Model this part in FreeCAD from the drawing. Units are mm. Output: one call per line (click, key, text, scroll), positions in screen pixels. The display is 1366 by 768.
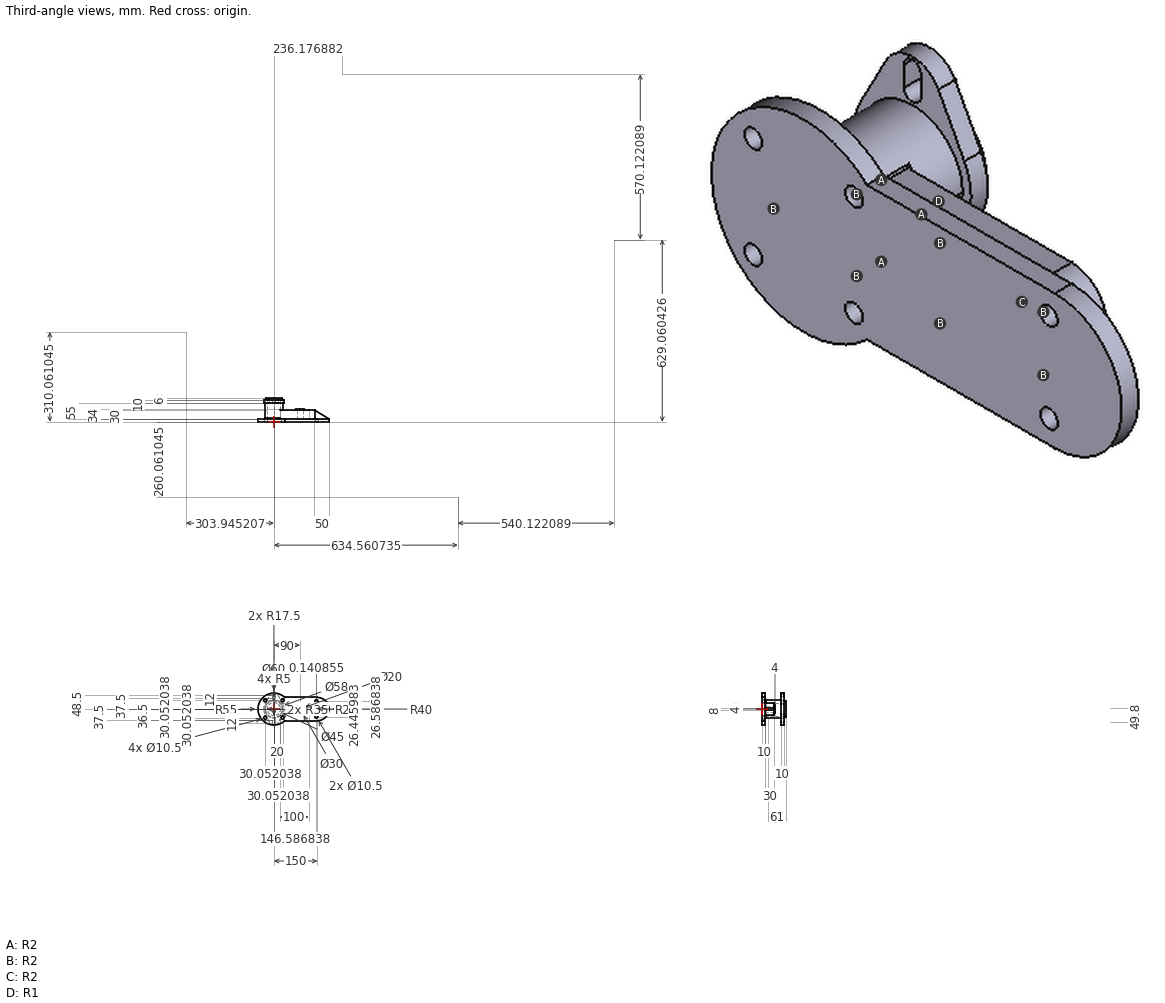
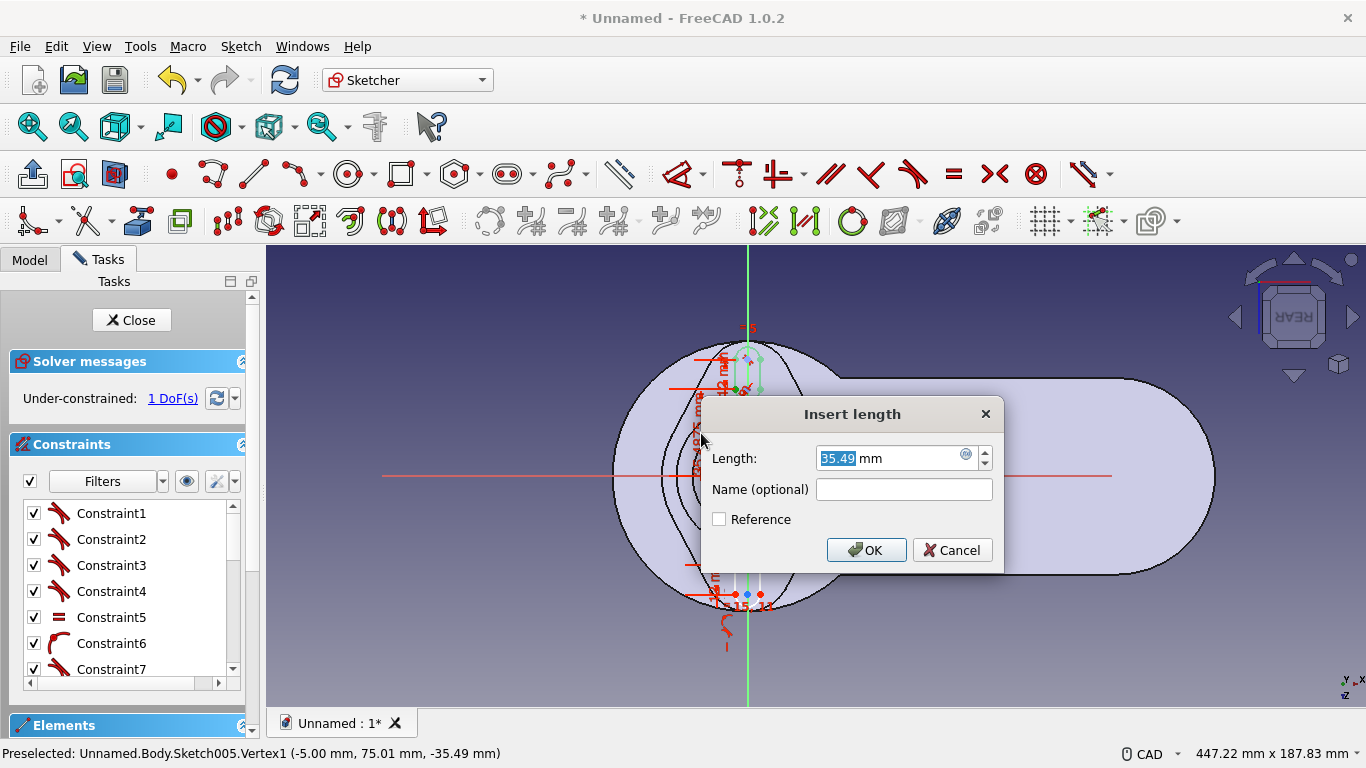
text(36.5)
key(Return)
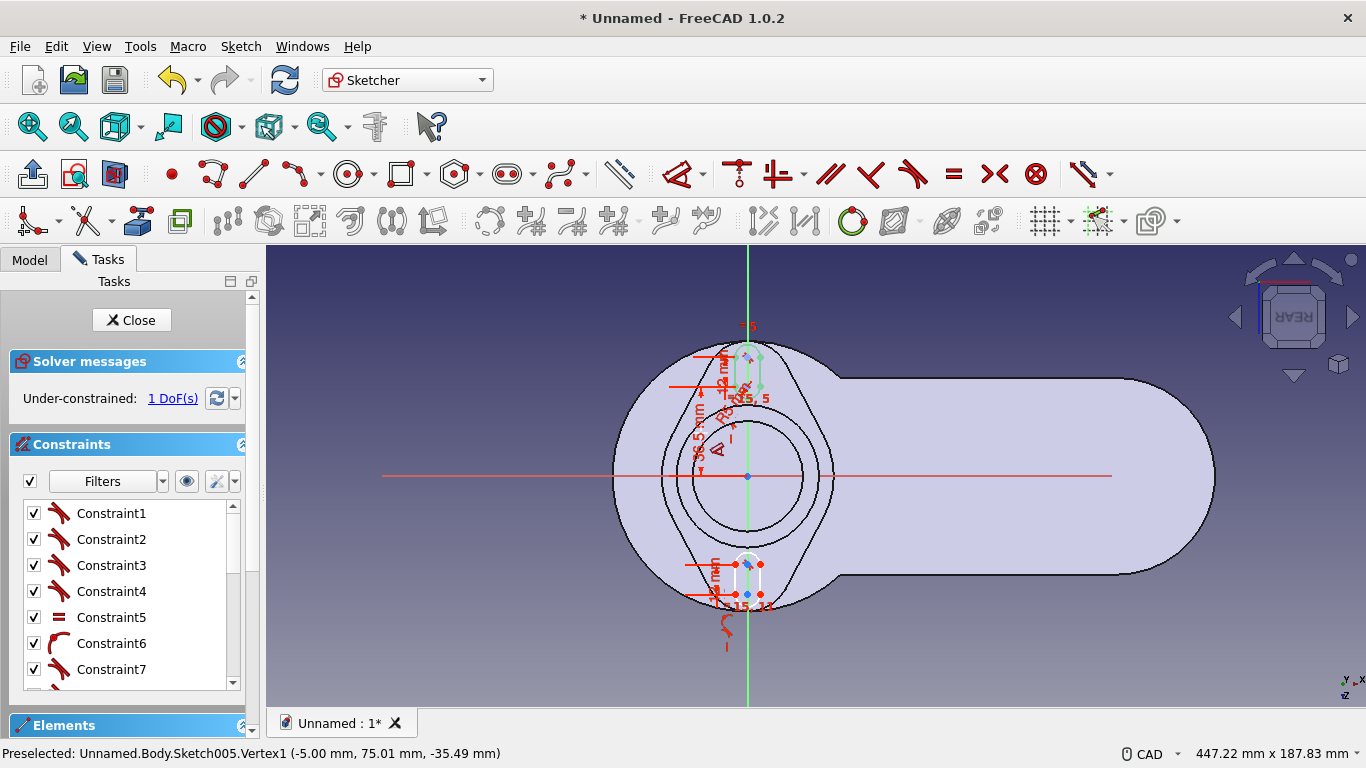
click(735, 595)
click(701, 535)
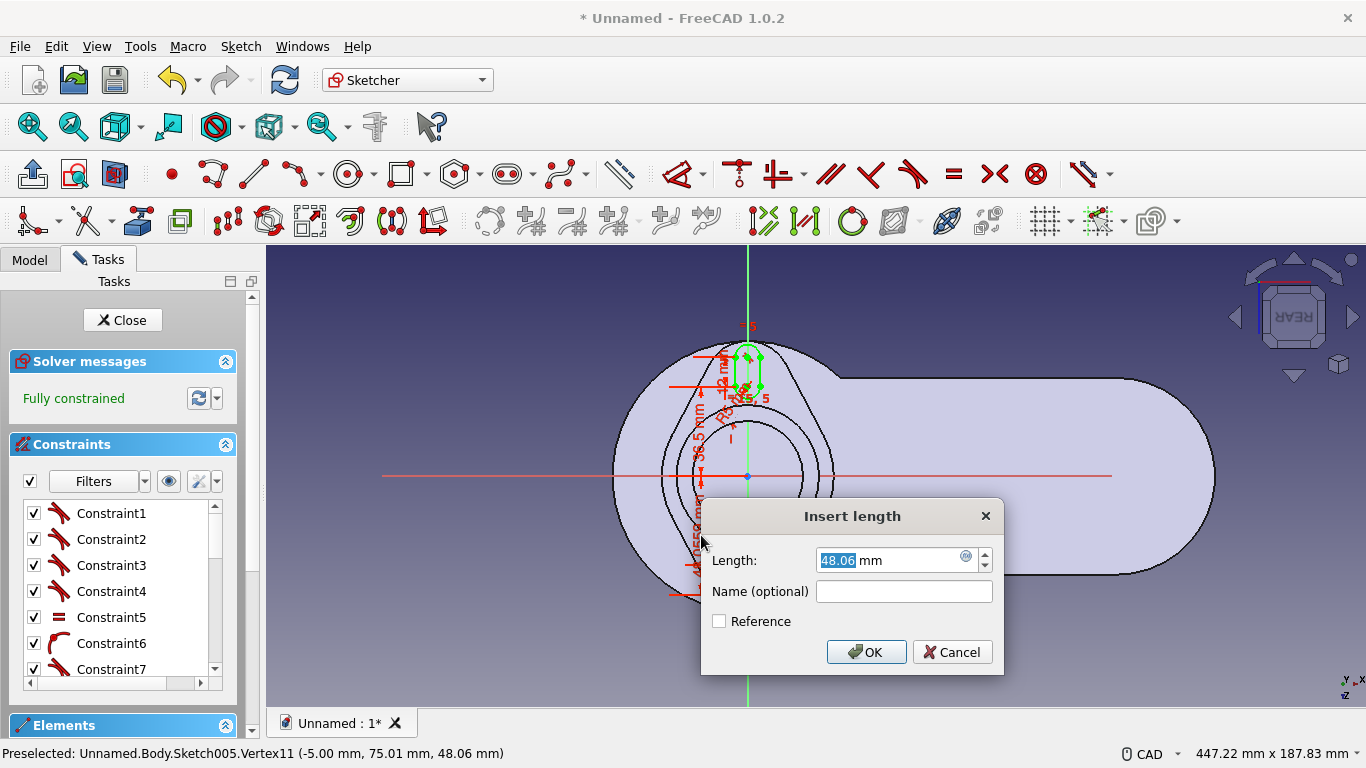
text(48.5)
key(Return)
key(Escape)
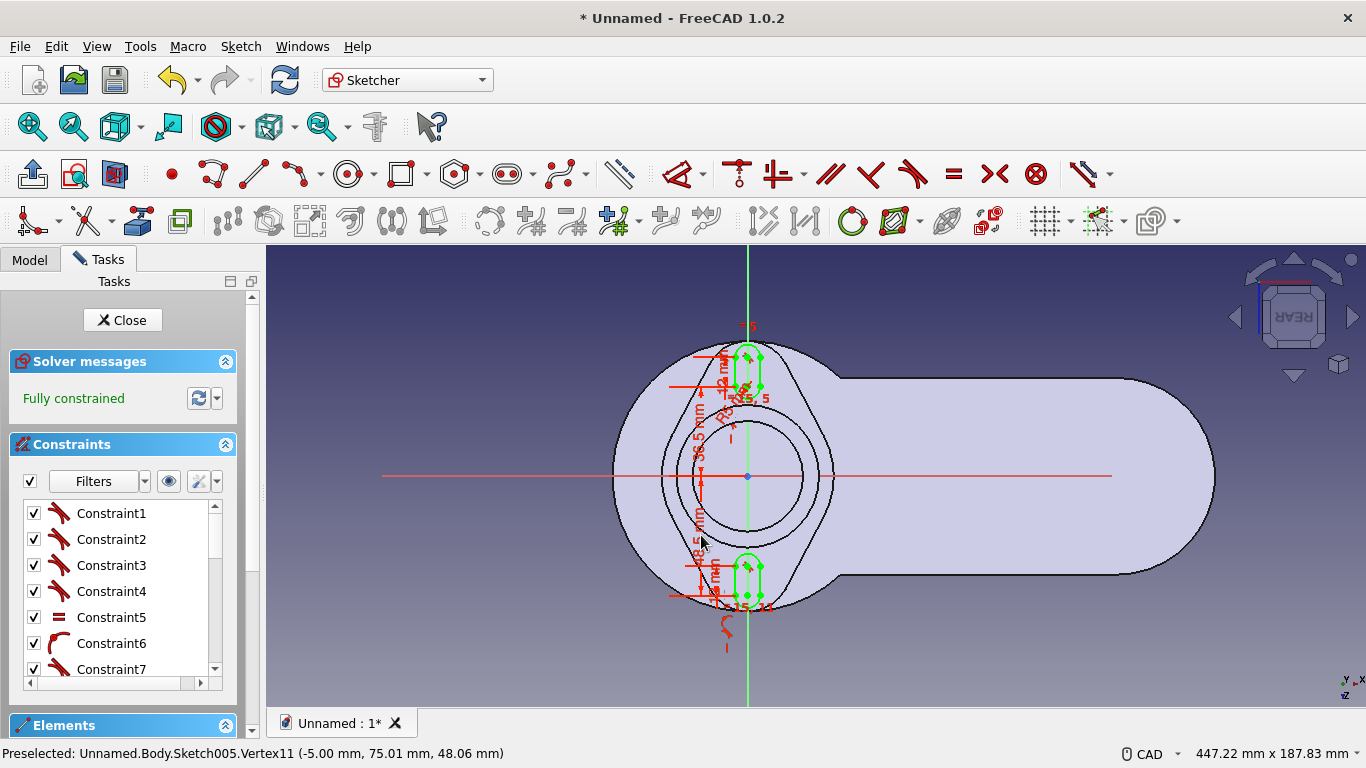
click(123, 320)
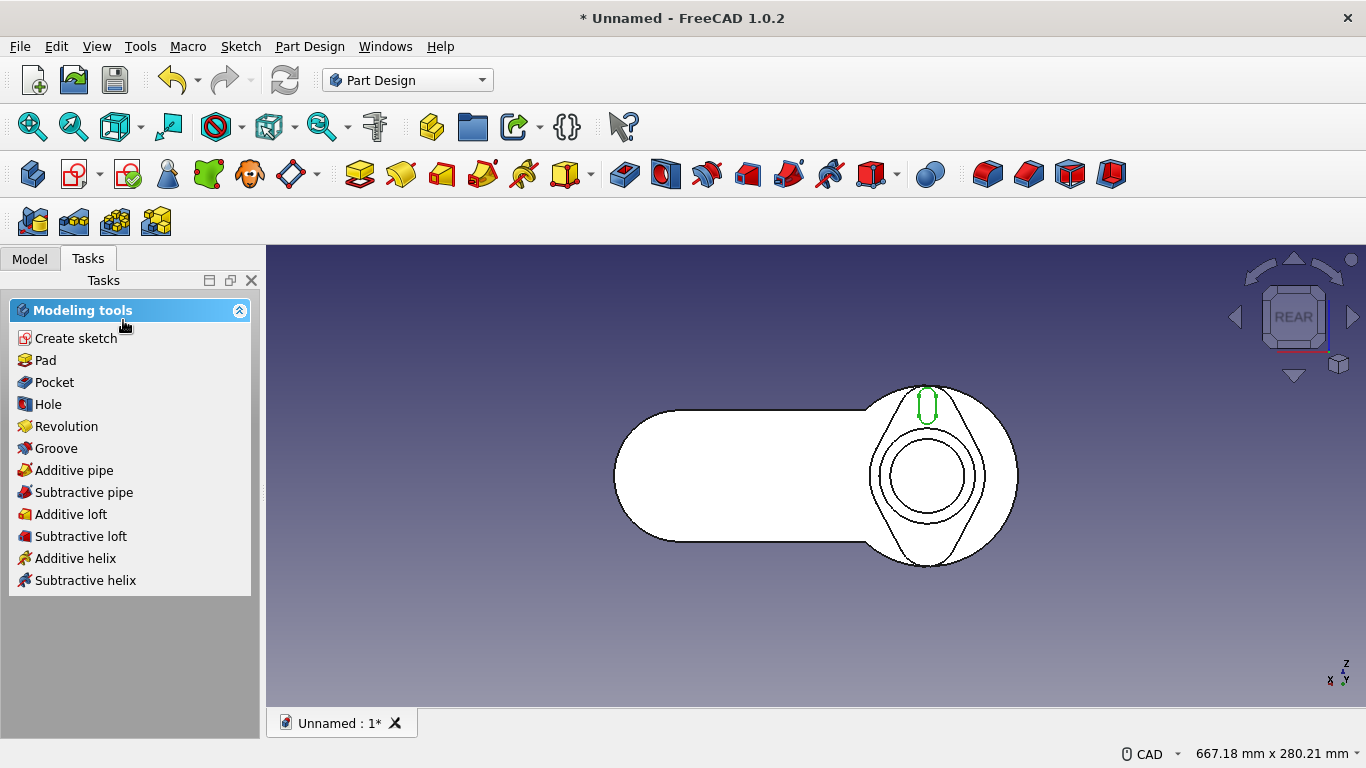
click(625, 174)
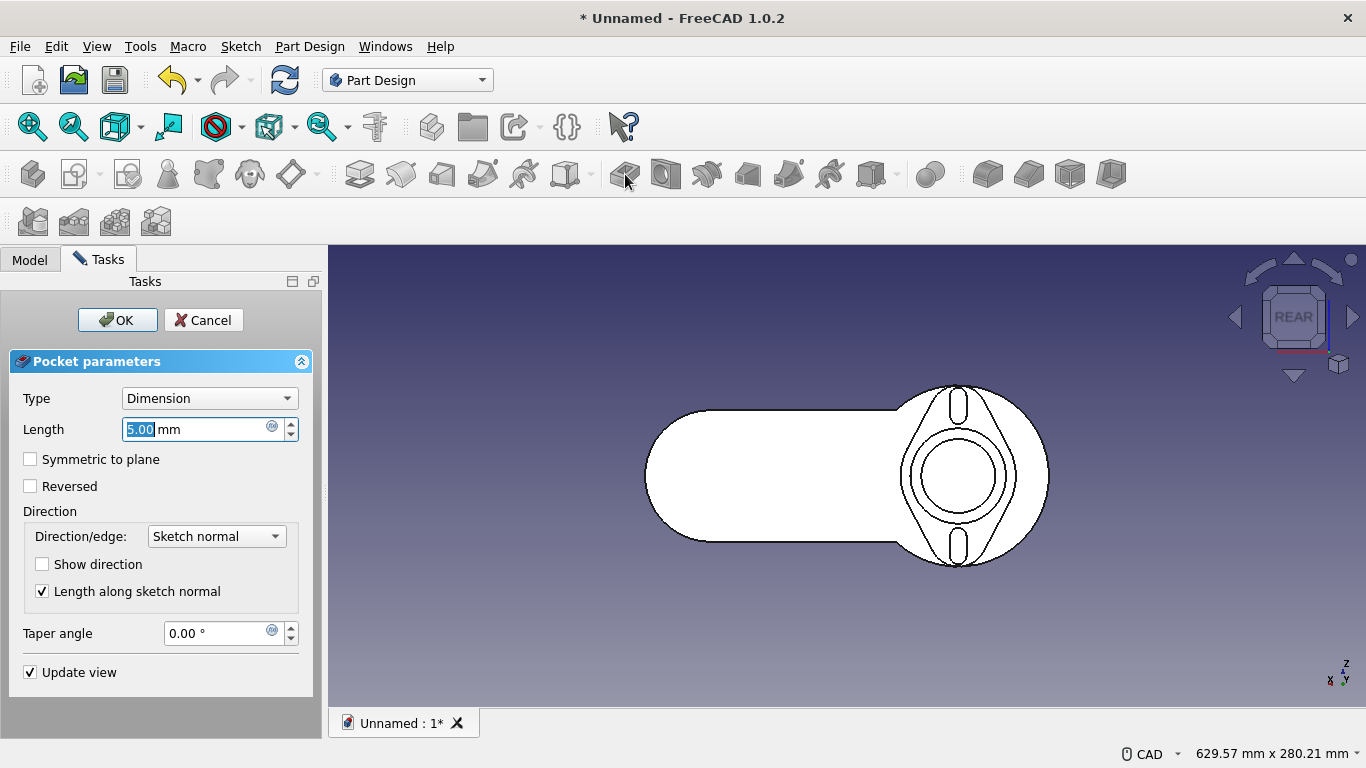
text(10)
key(Tab)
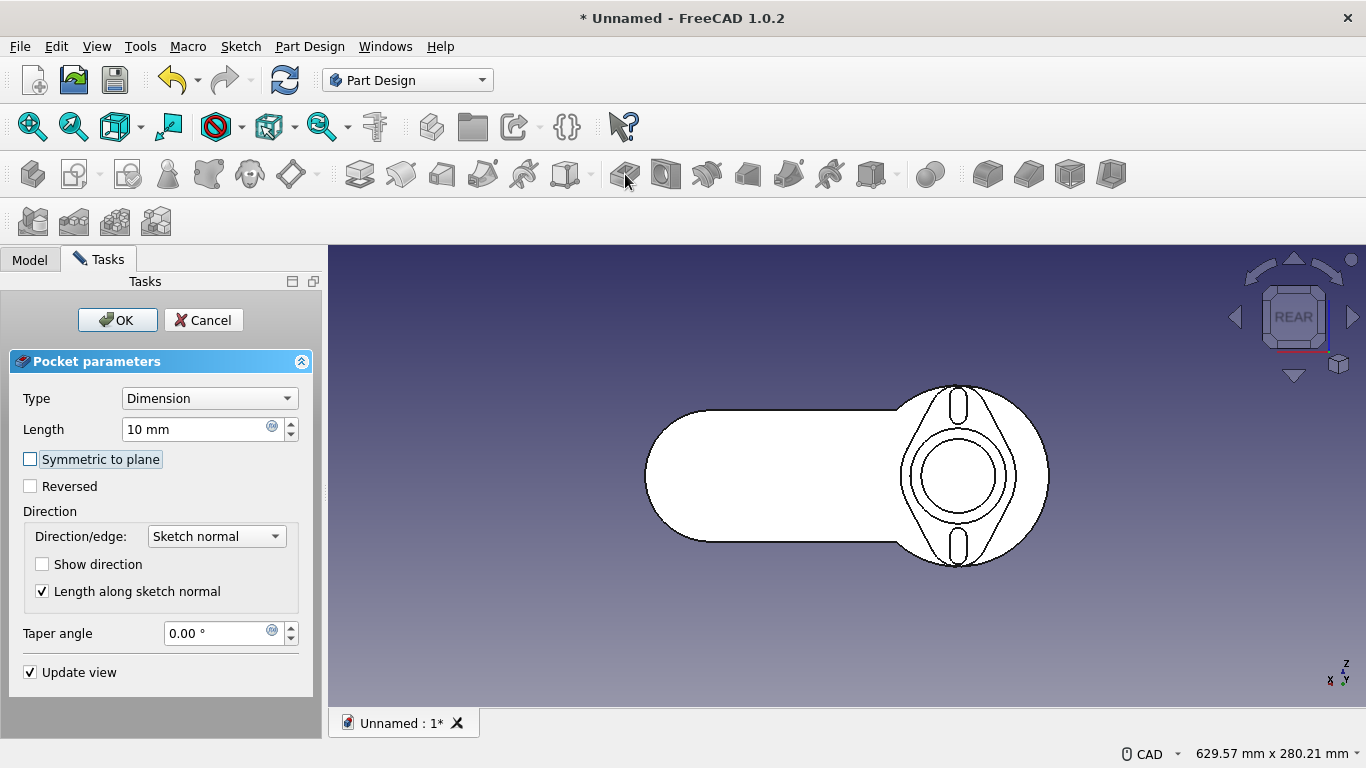
click(118, 320)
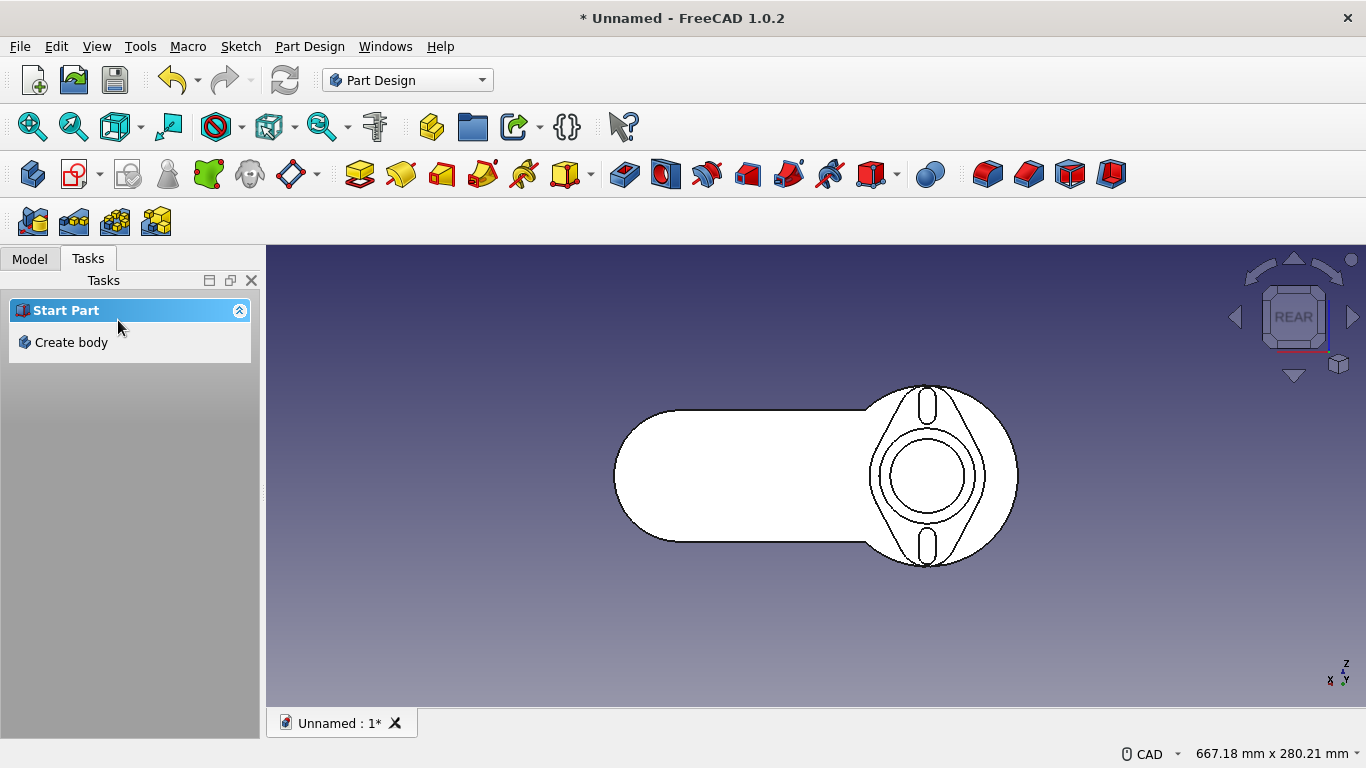
click(33, 128)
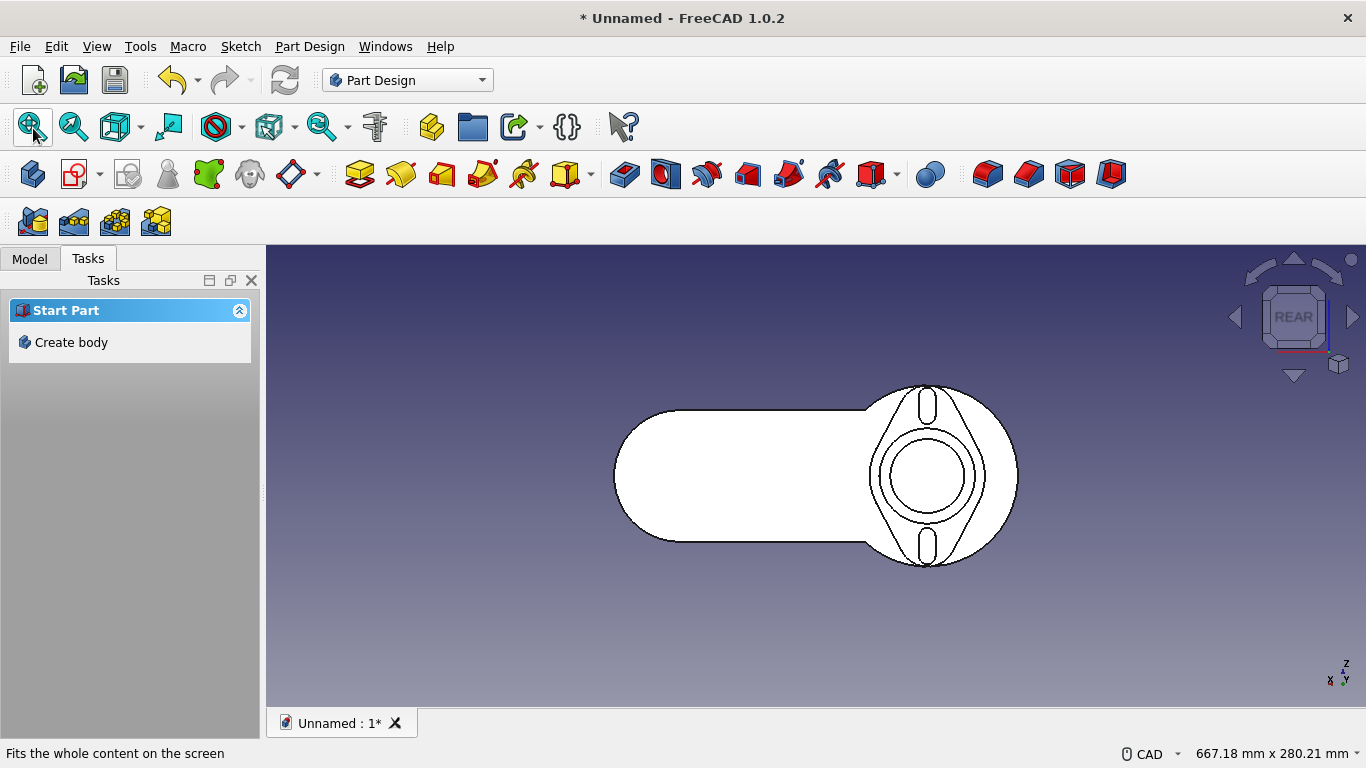
click(701, 475)